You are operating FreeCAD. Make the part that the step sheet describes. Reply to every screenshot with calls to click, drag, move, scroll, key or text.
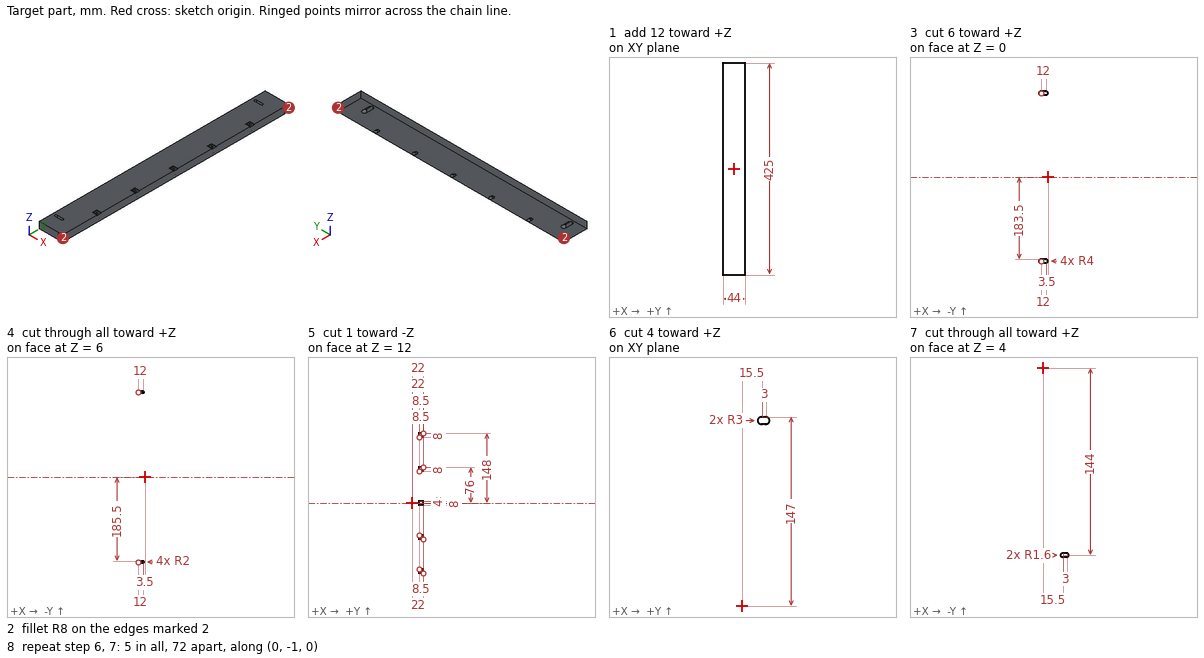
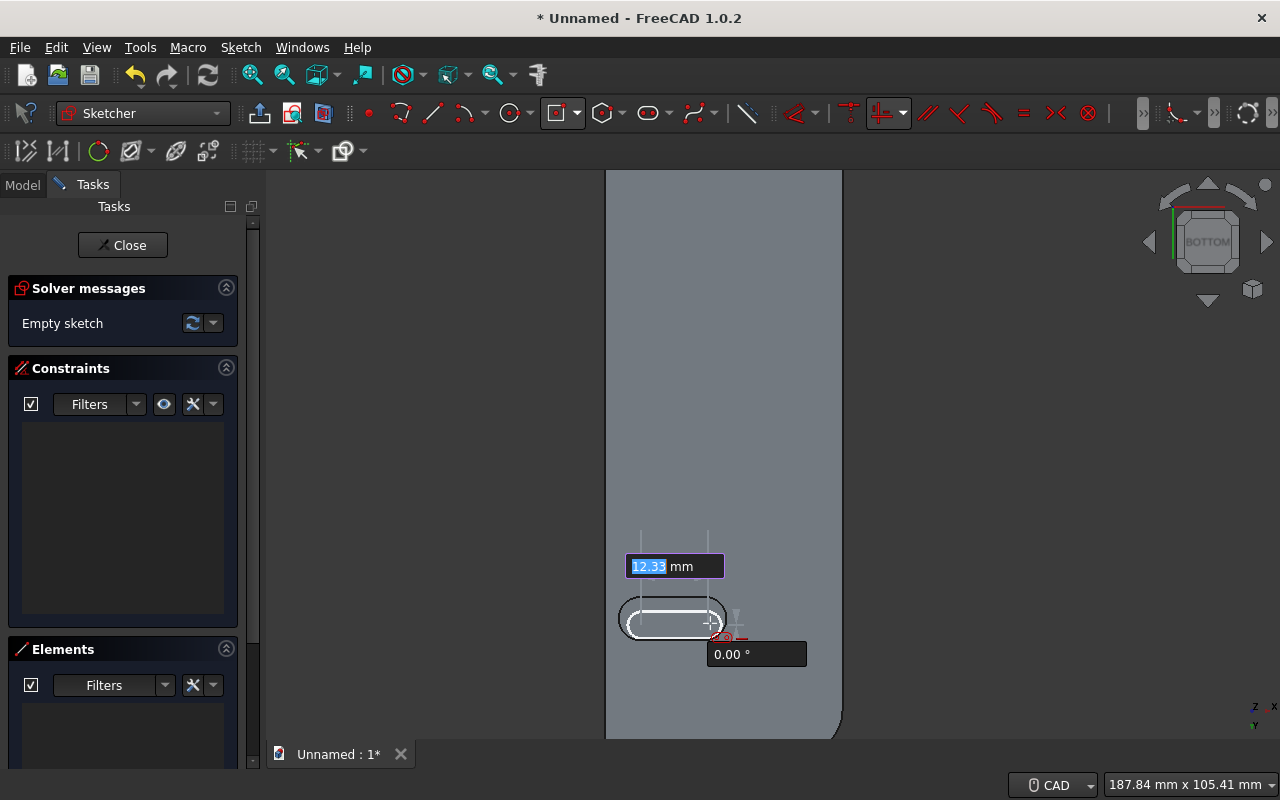
click(705, 619)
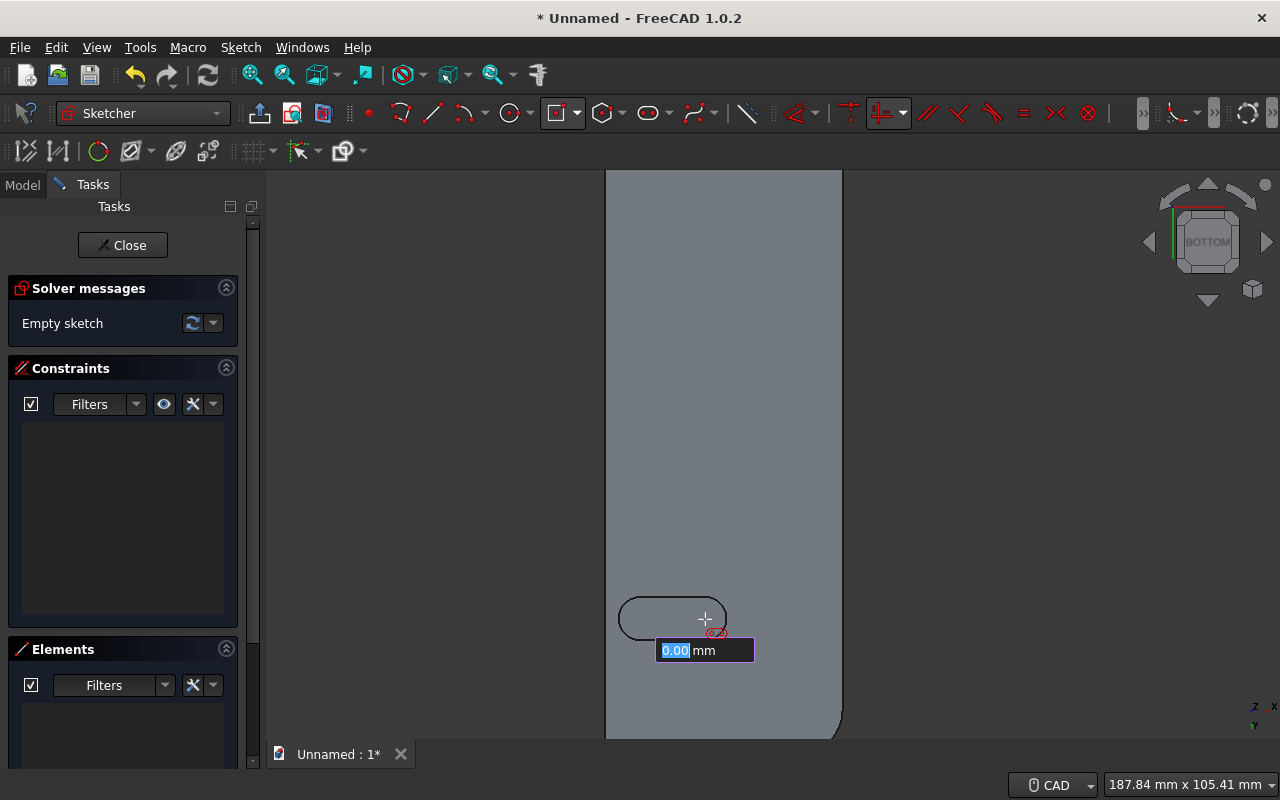
scroll(673, 629, up, 2)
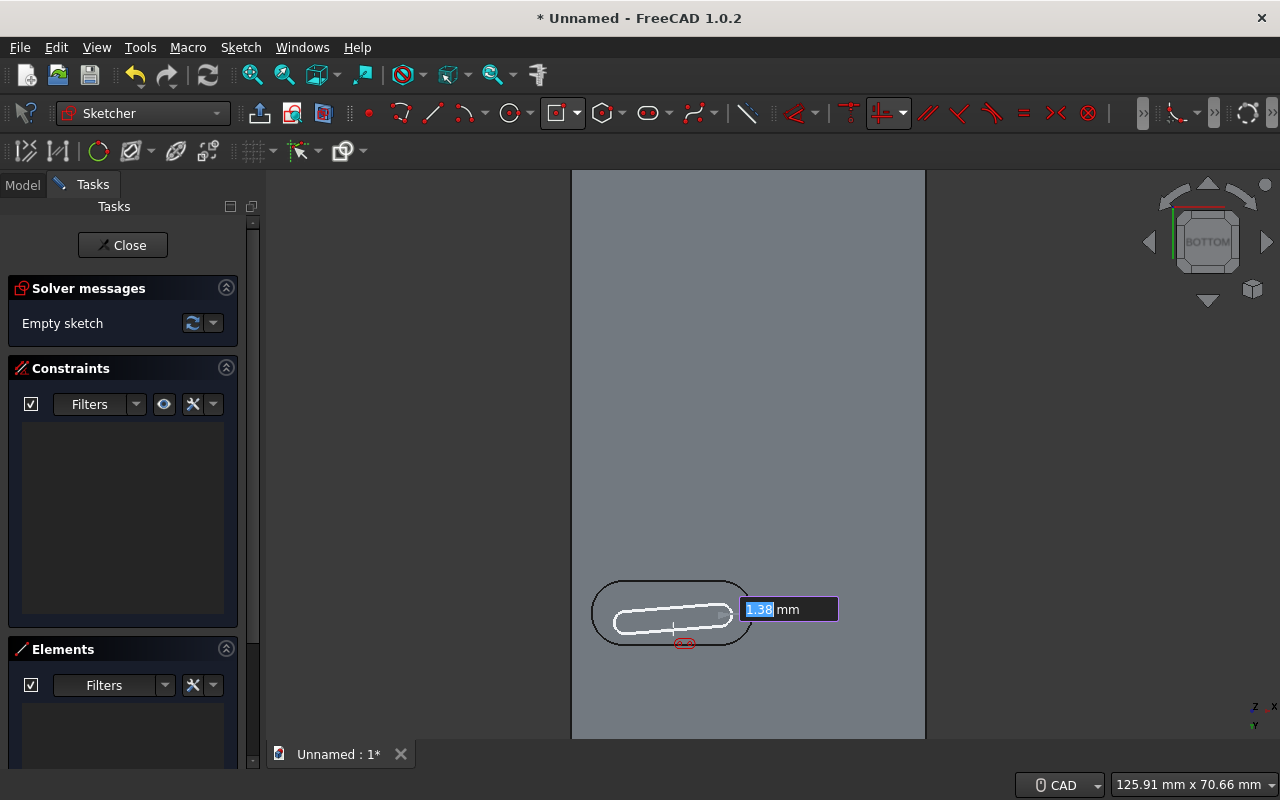
click(672, 629)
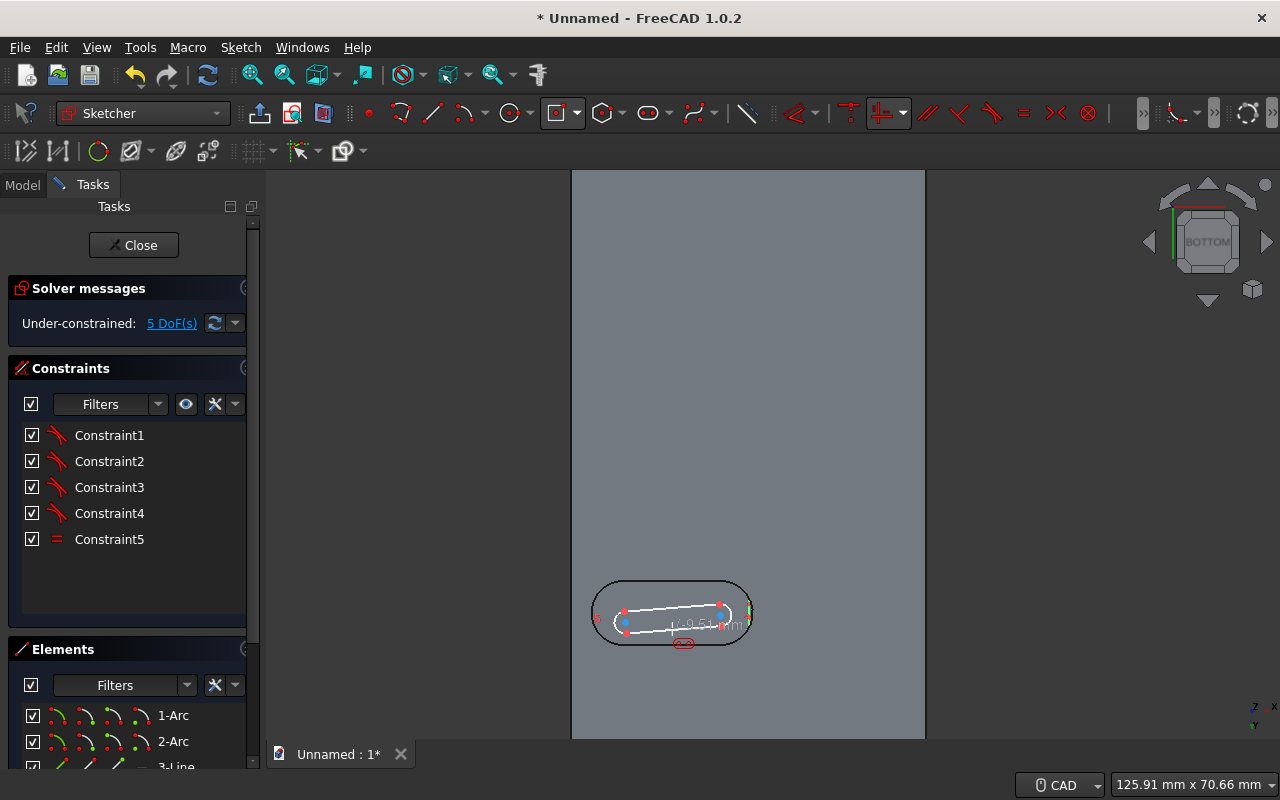
scroll(708, 623, down, 11)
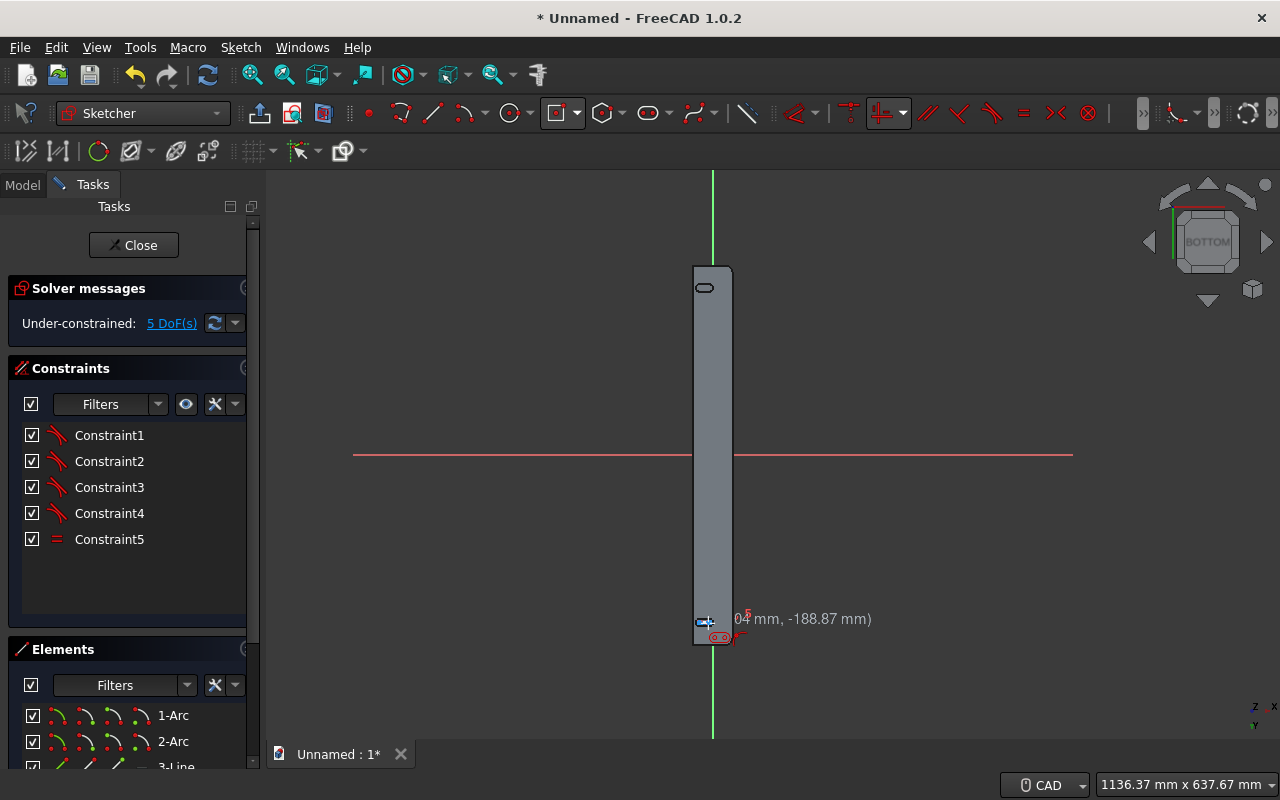
scroll(699, 288, up, 13)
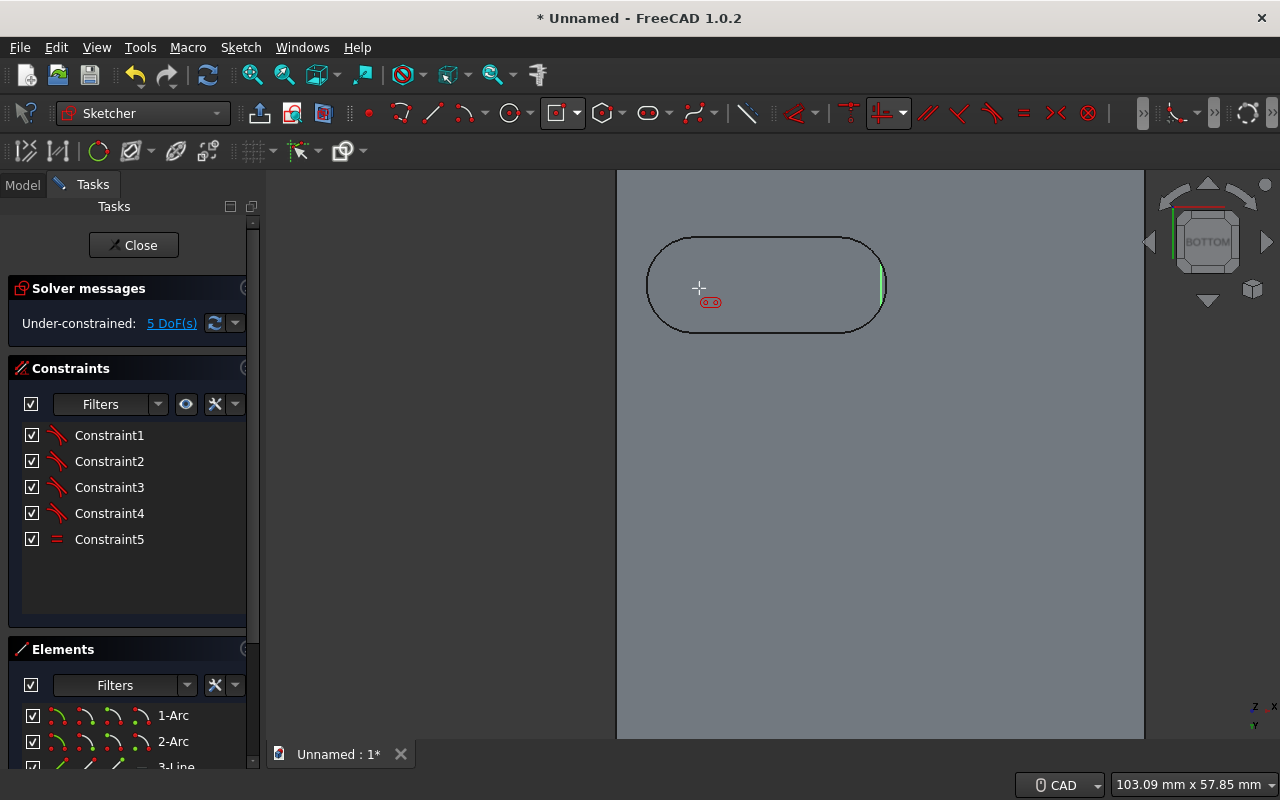
scroll(699, 287, down, 13)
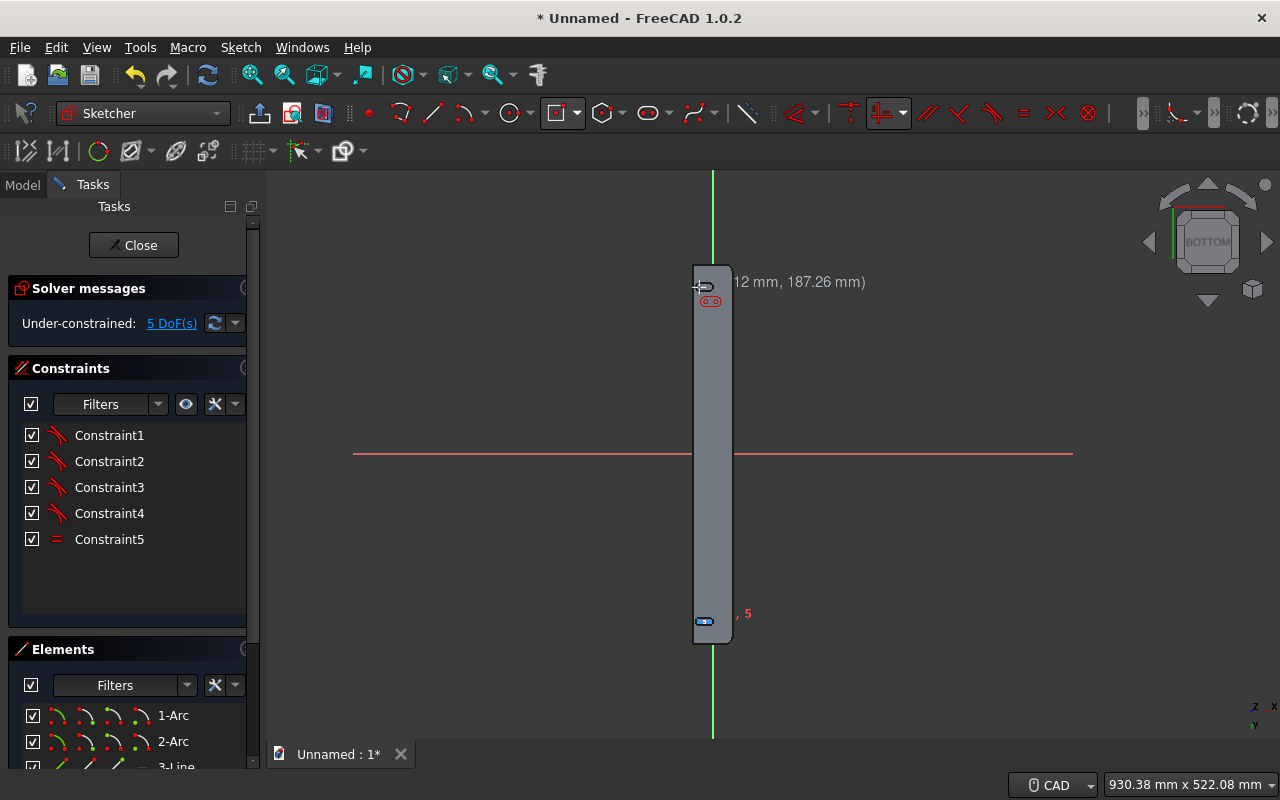
click(699, 287)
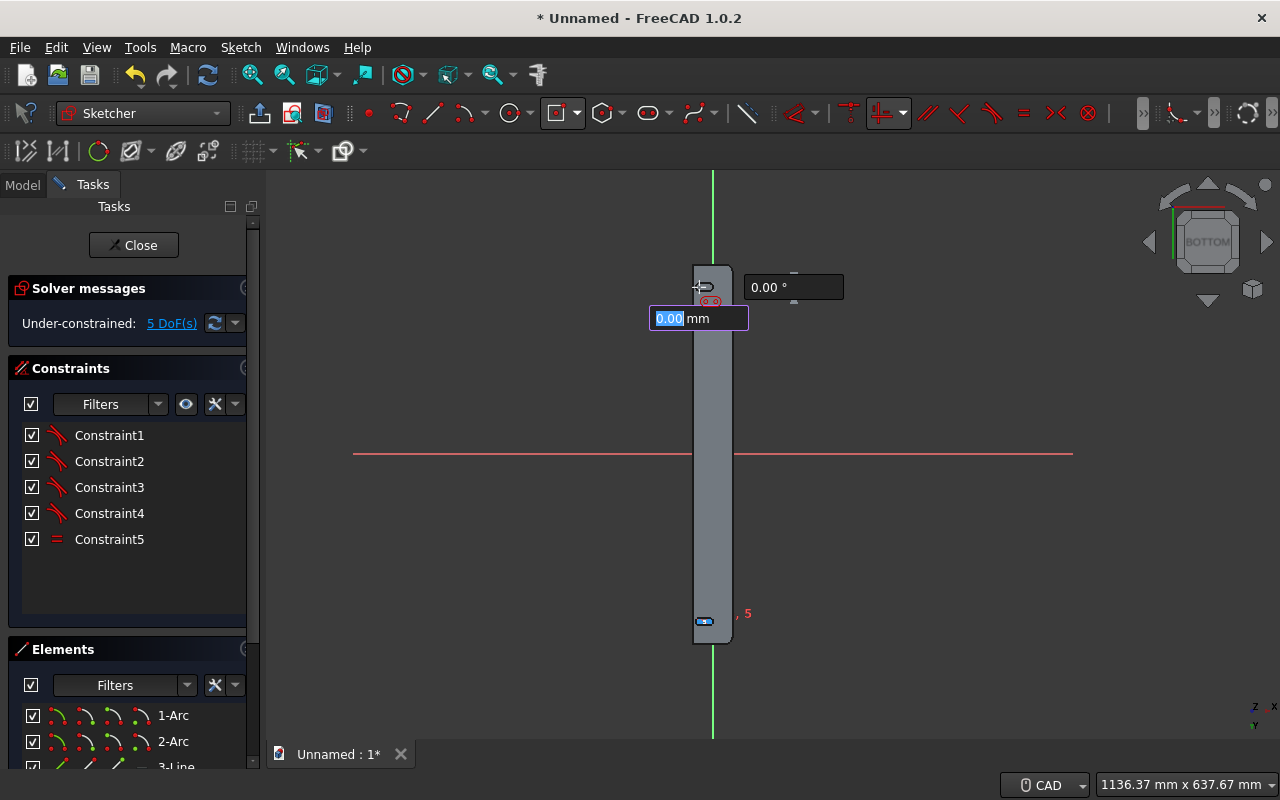
scroll(710, 287, up, 9)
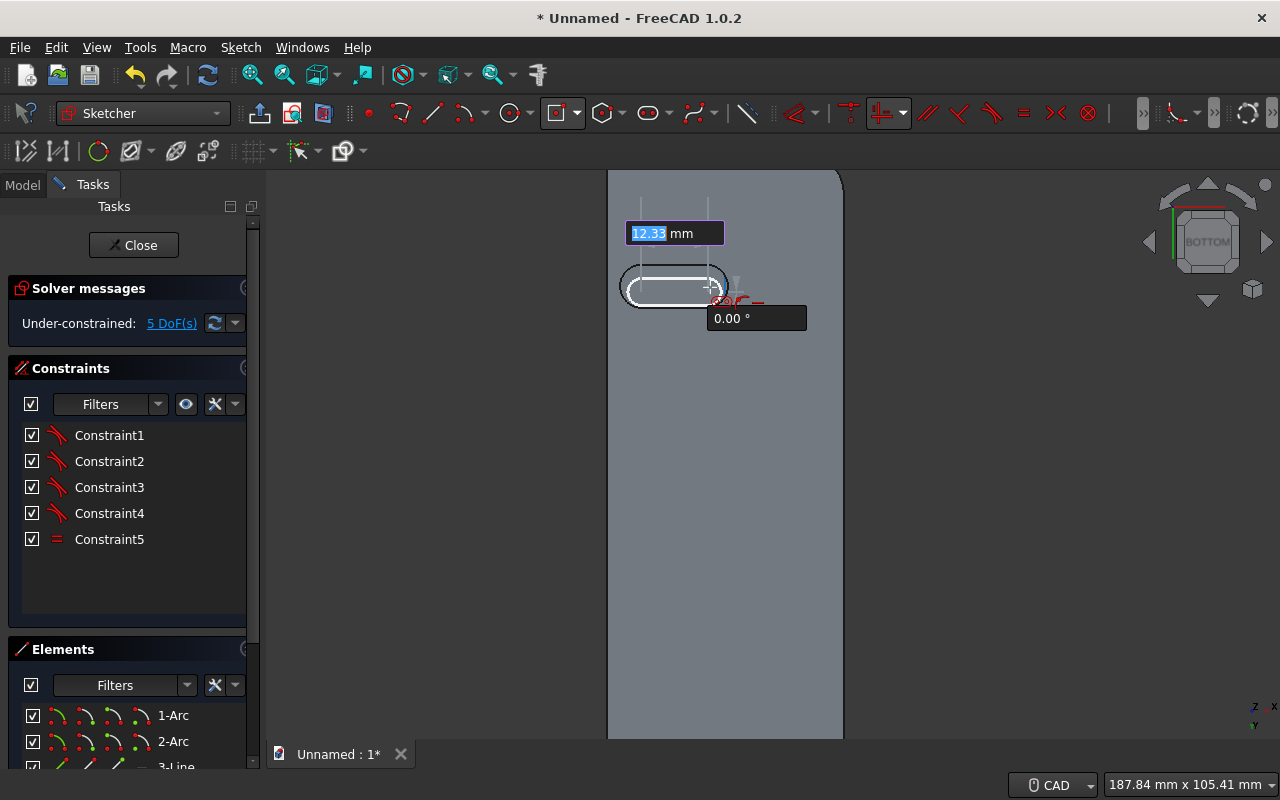
click(706, 286)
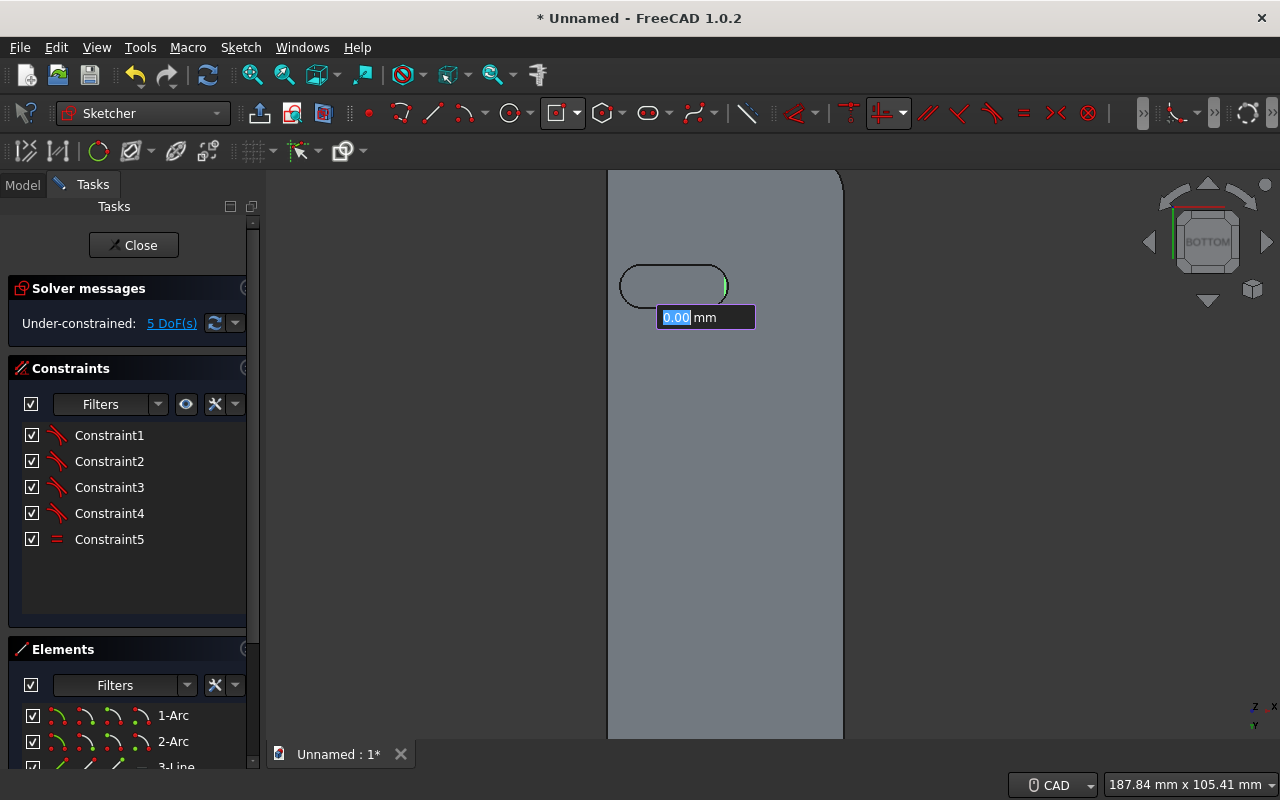
scroll(674, 275, up, 2)